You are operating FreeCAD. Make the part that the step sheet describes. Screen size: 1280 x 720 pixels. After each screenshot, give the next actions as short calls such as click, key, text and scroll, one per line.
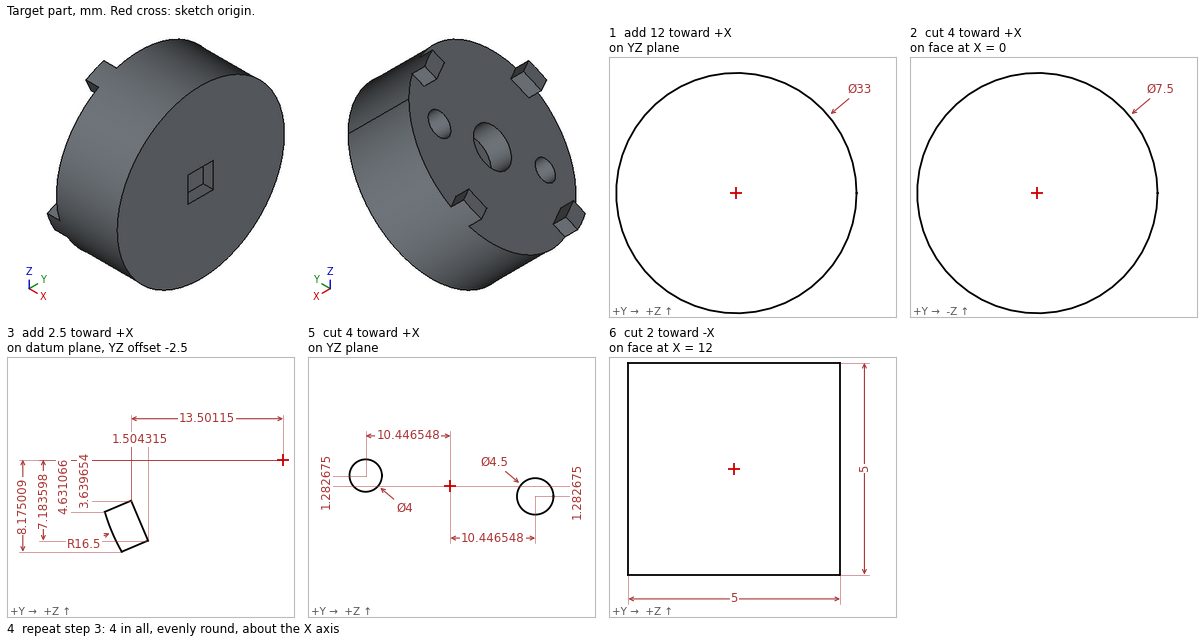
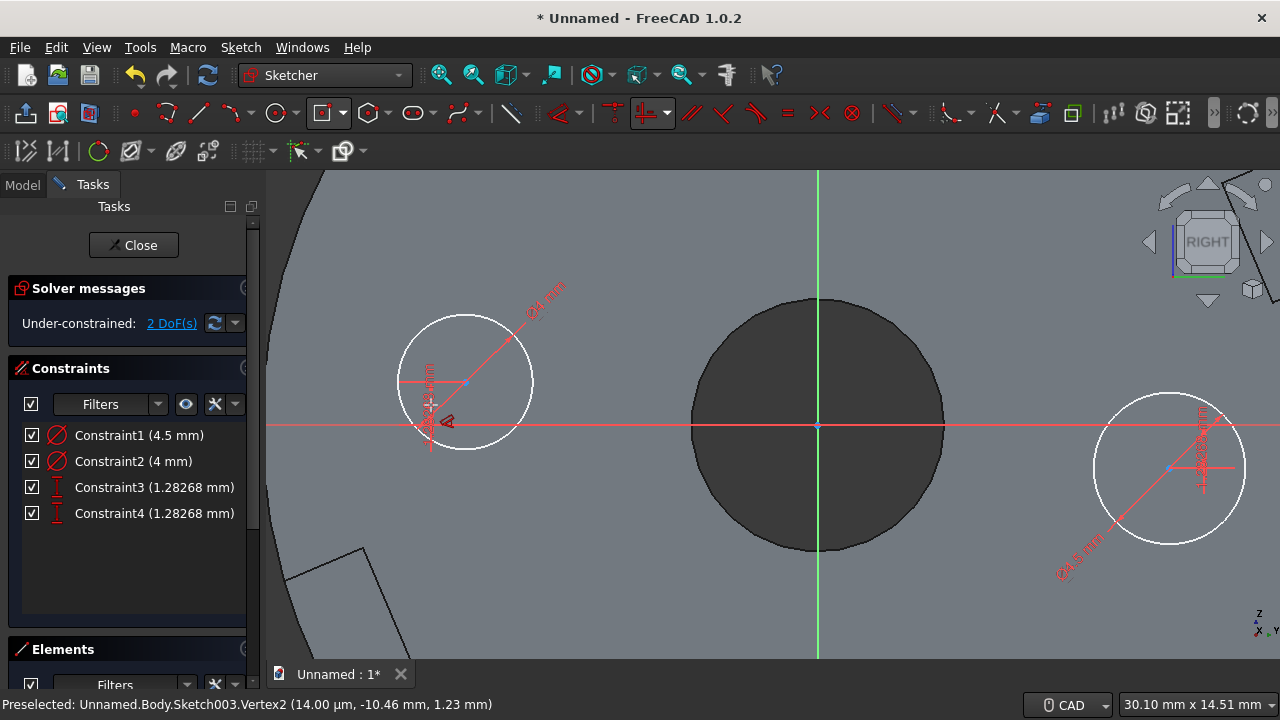
scroll(466, 384, down, 2)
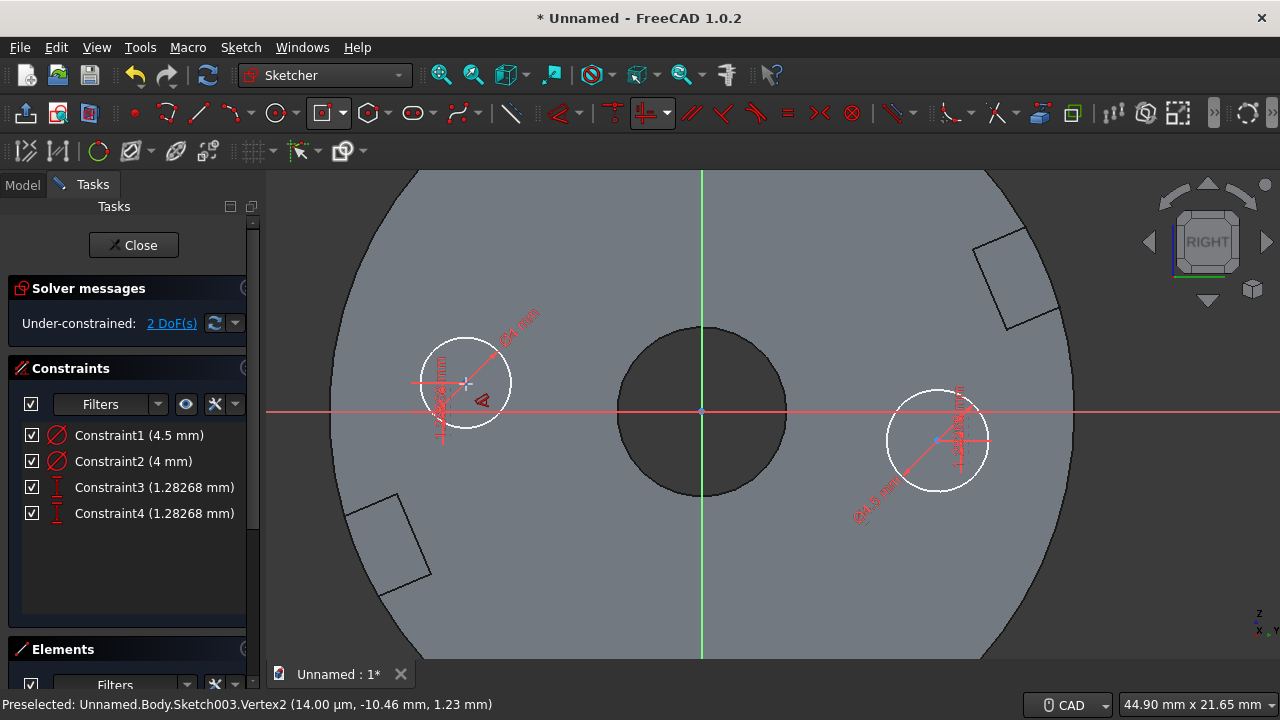
click(938, 441)
click(820, 475)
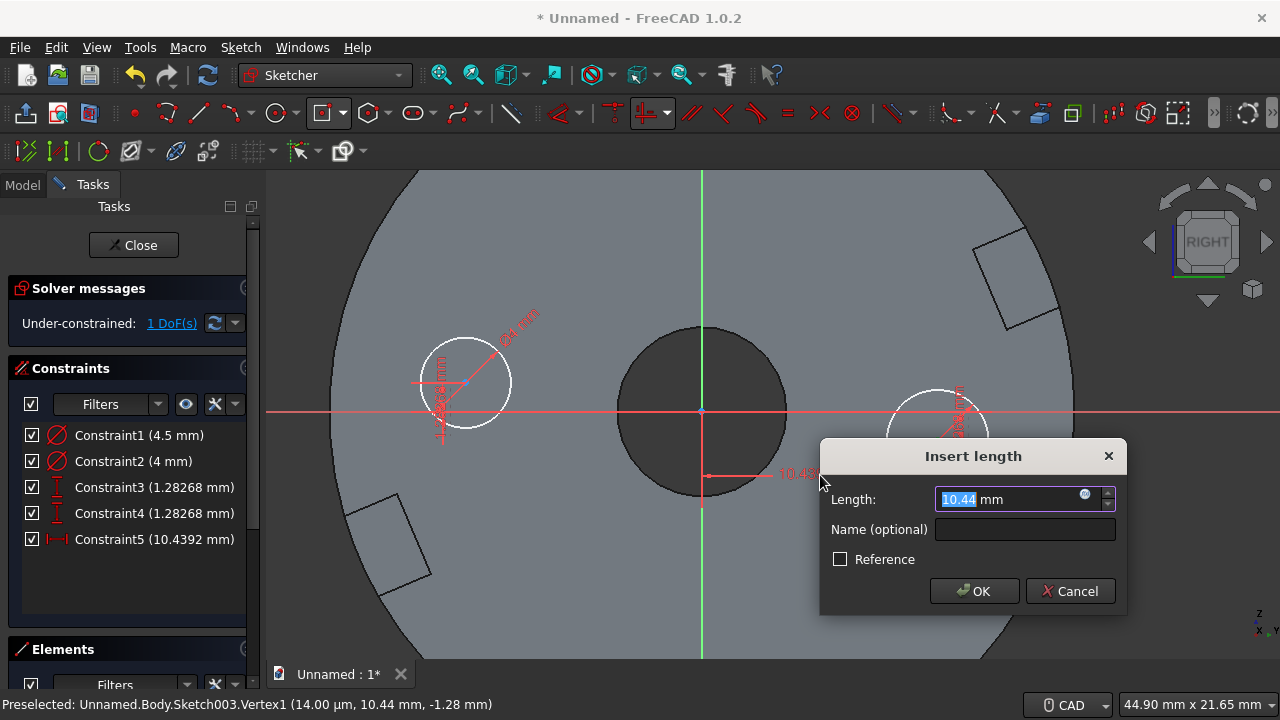
text(10.446548)
key(Return)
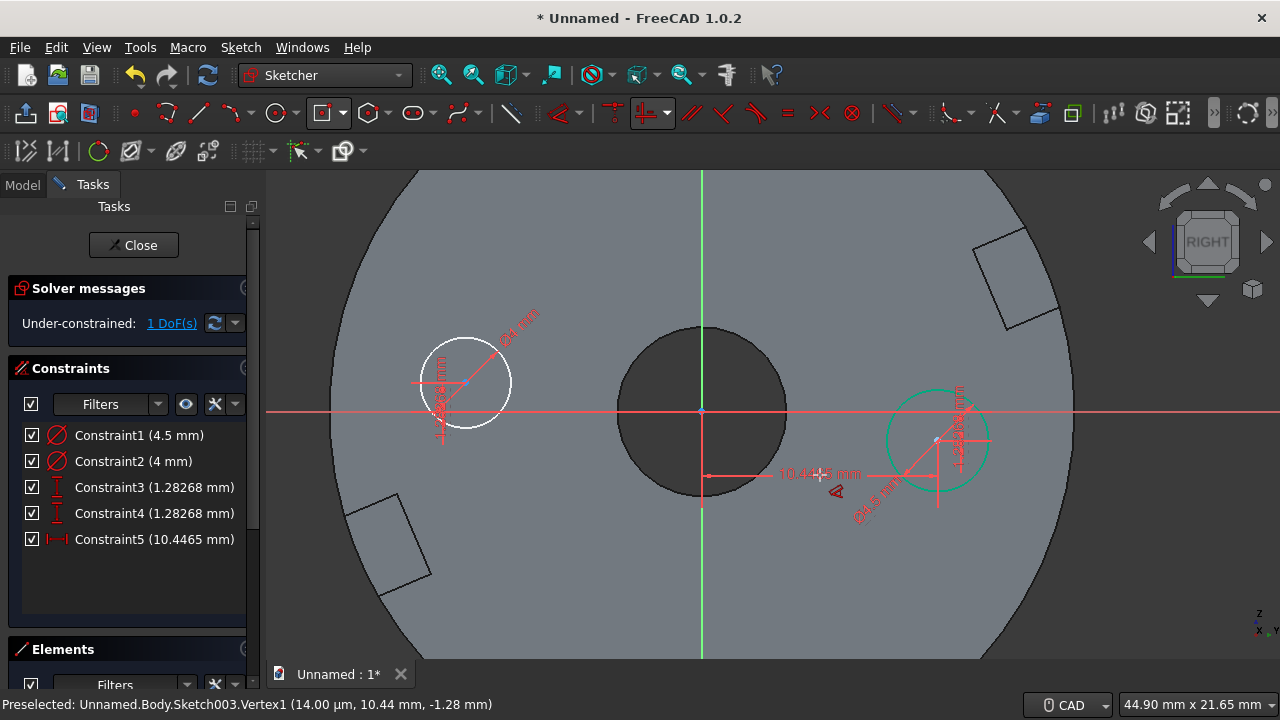
click(466, 383)
click(638, 349)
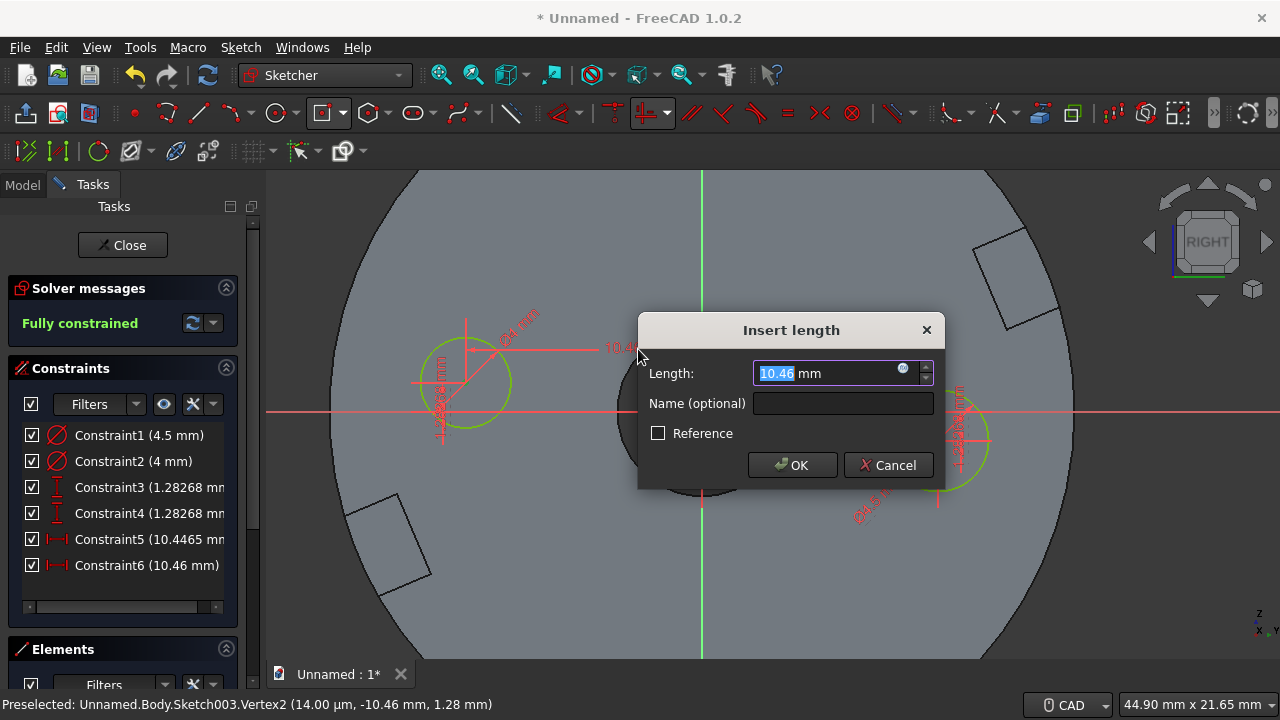
text(10.446548)
key(Return)
key(Escape)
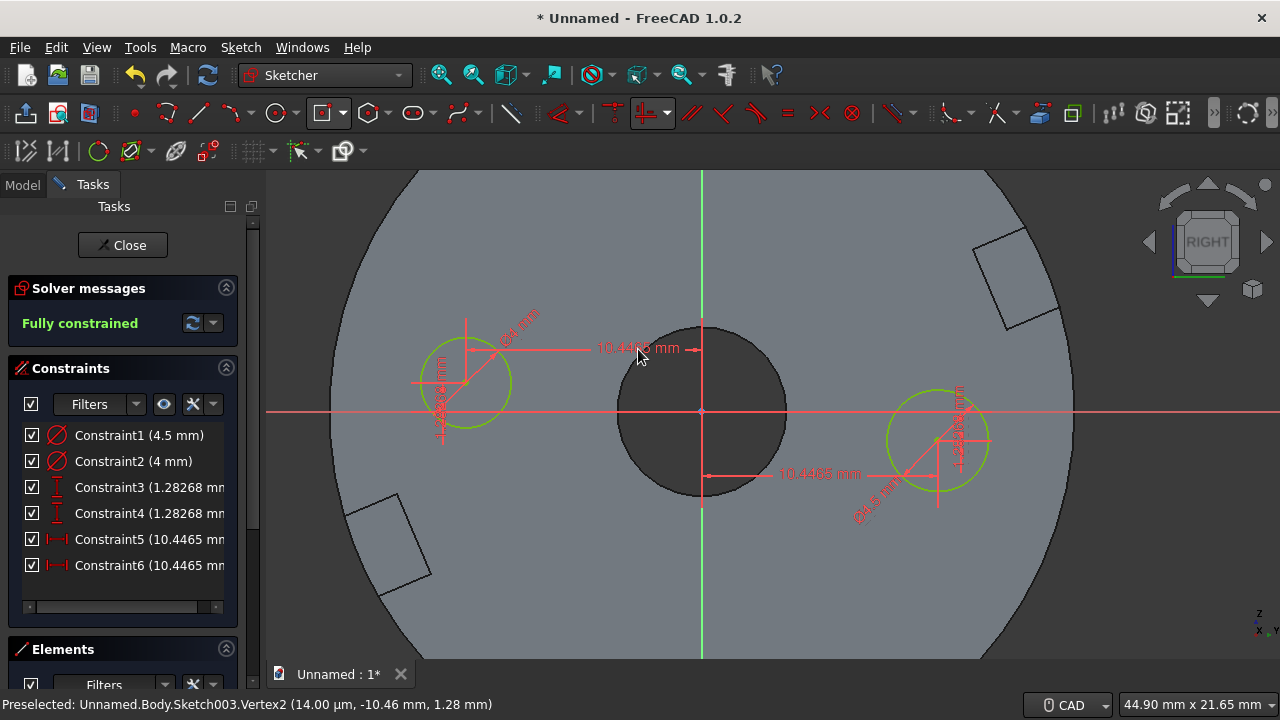
click(123, 245)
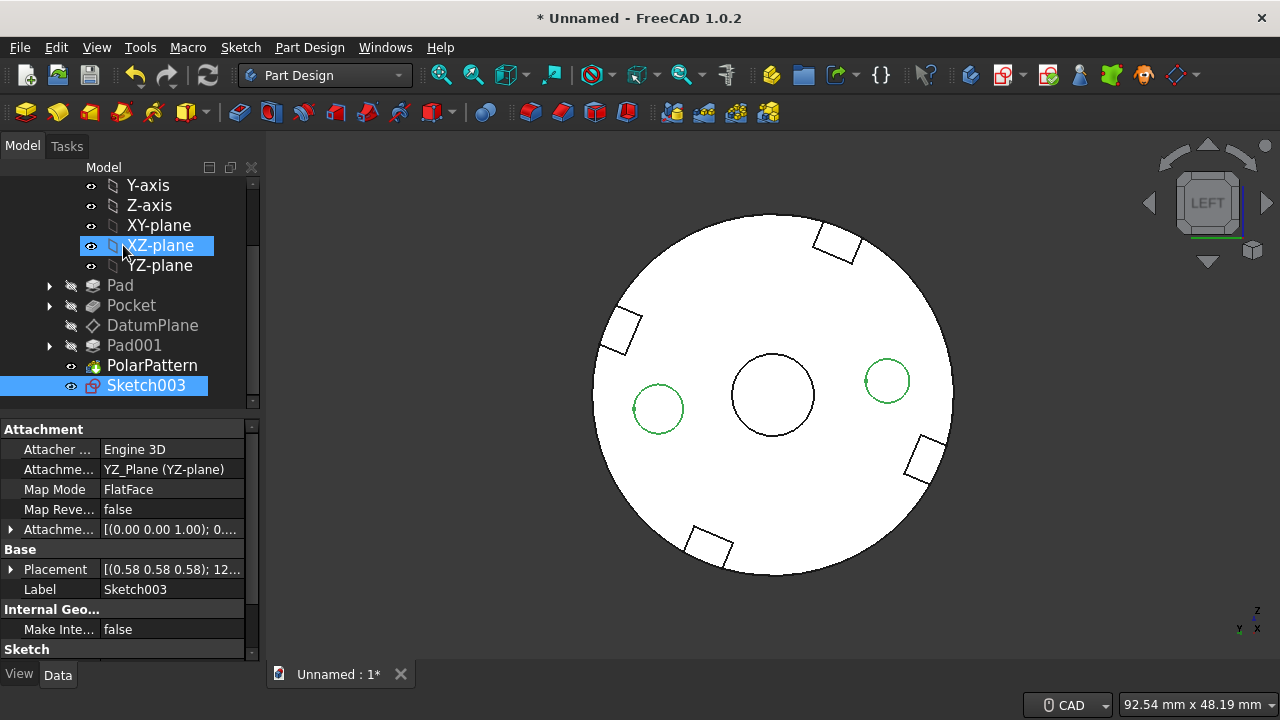
click(240, 112)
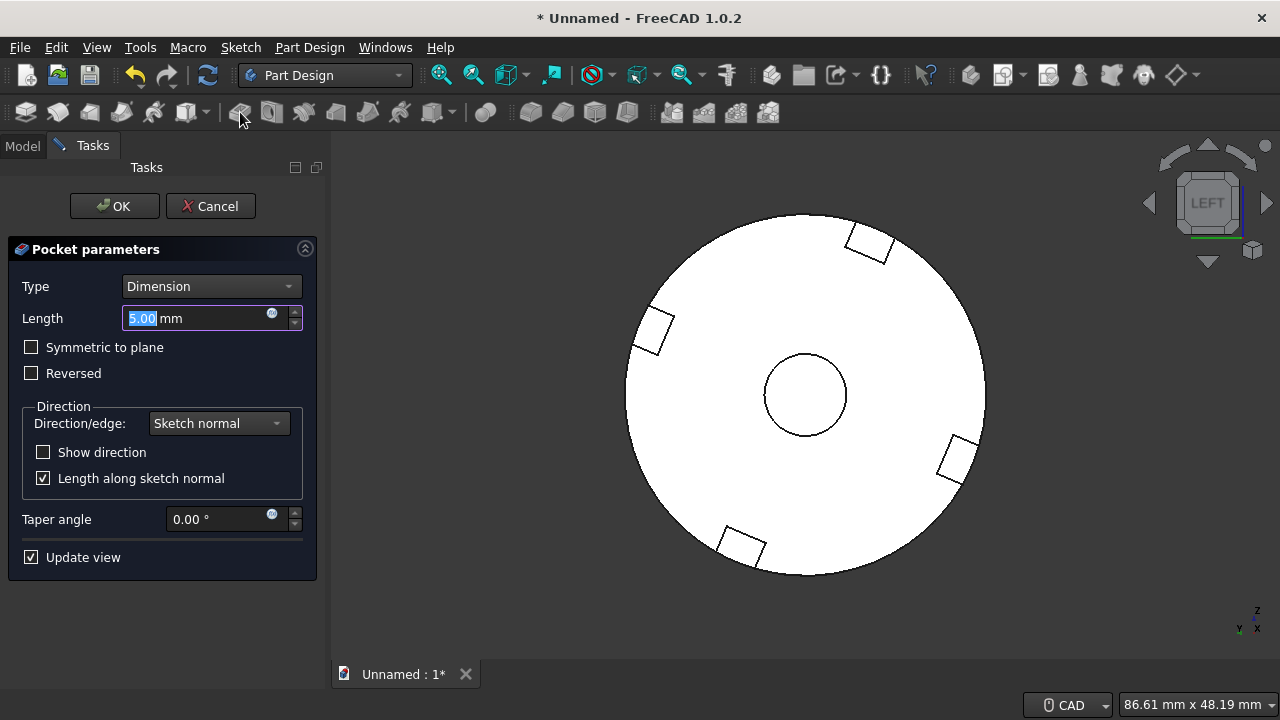
text(4)
key(Tab)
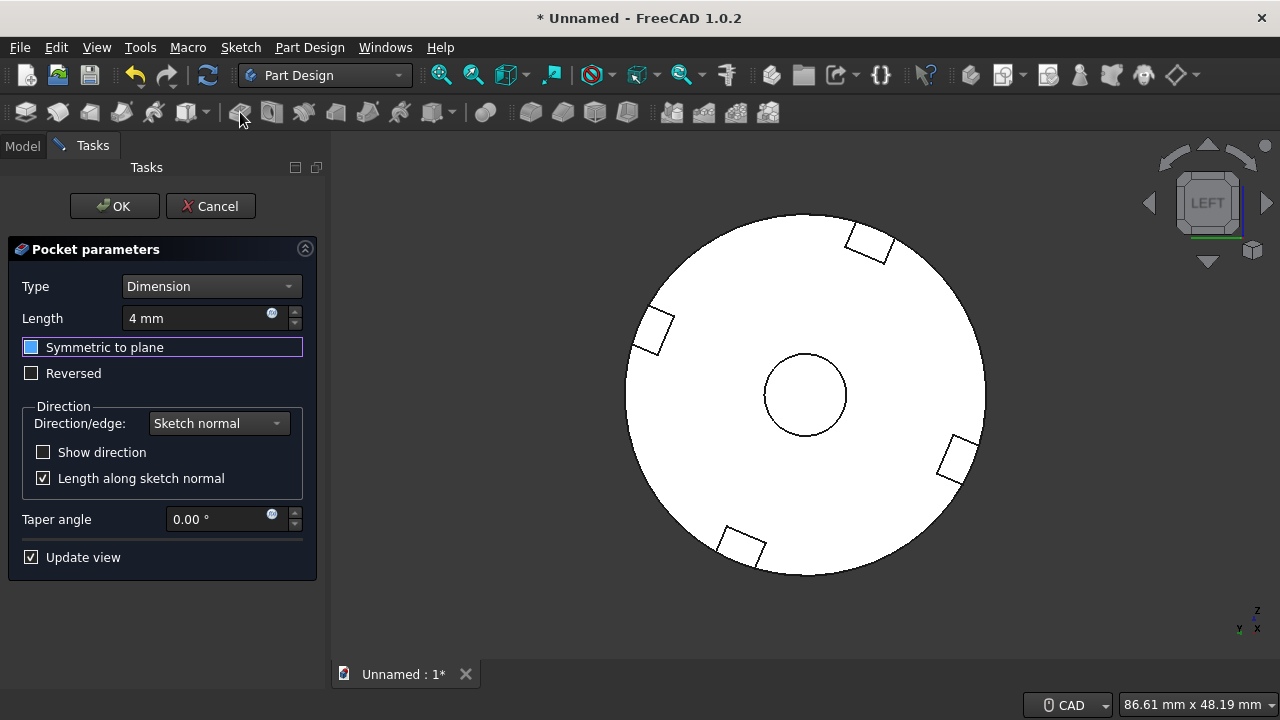
click(30, 373)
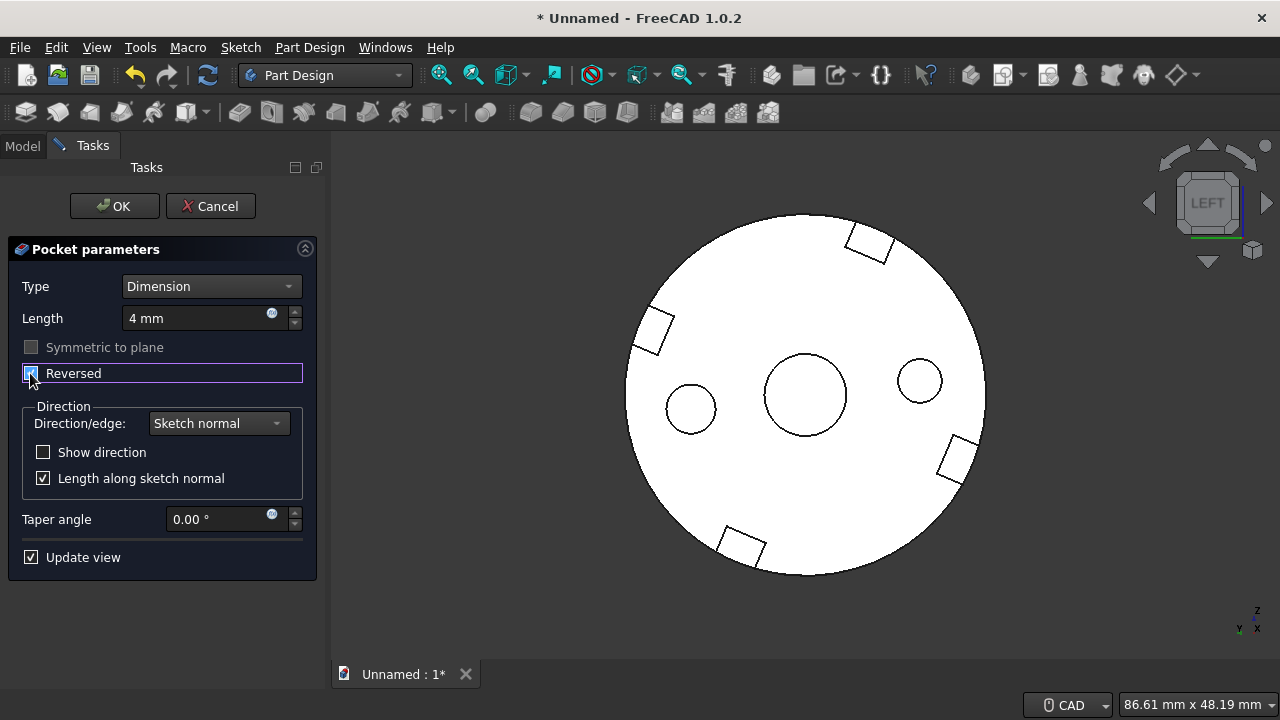
click(115, 206)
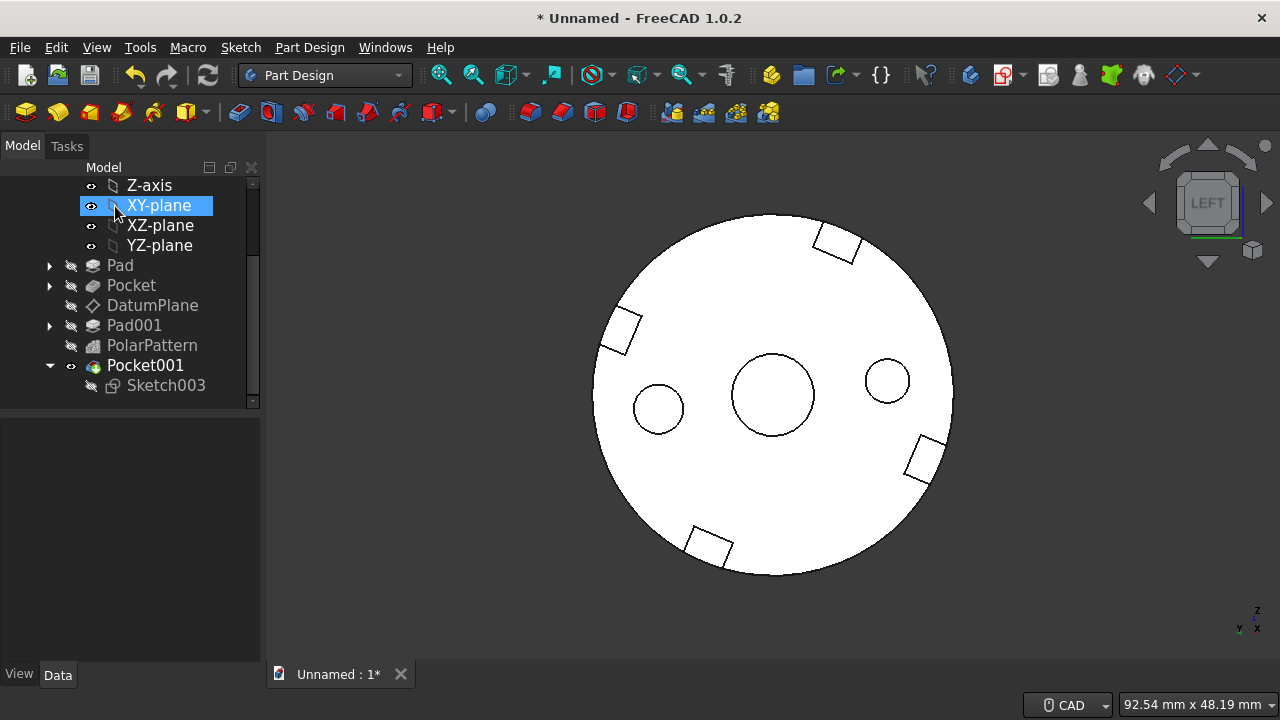
key(0)